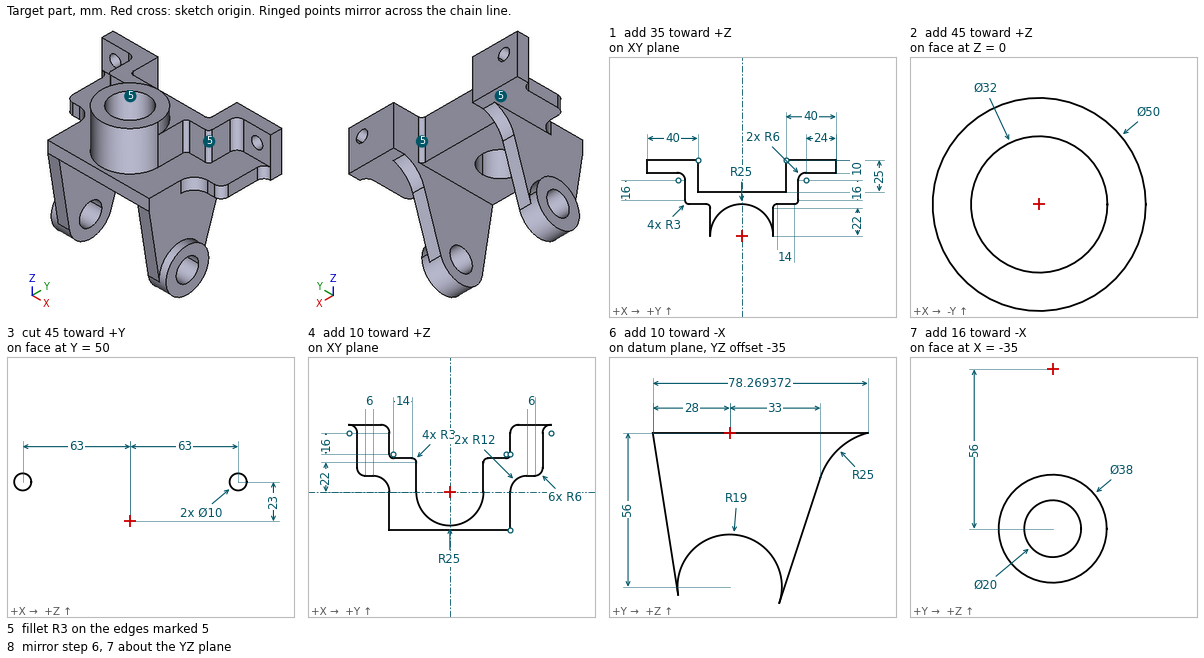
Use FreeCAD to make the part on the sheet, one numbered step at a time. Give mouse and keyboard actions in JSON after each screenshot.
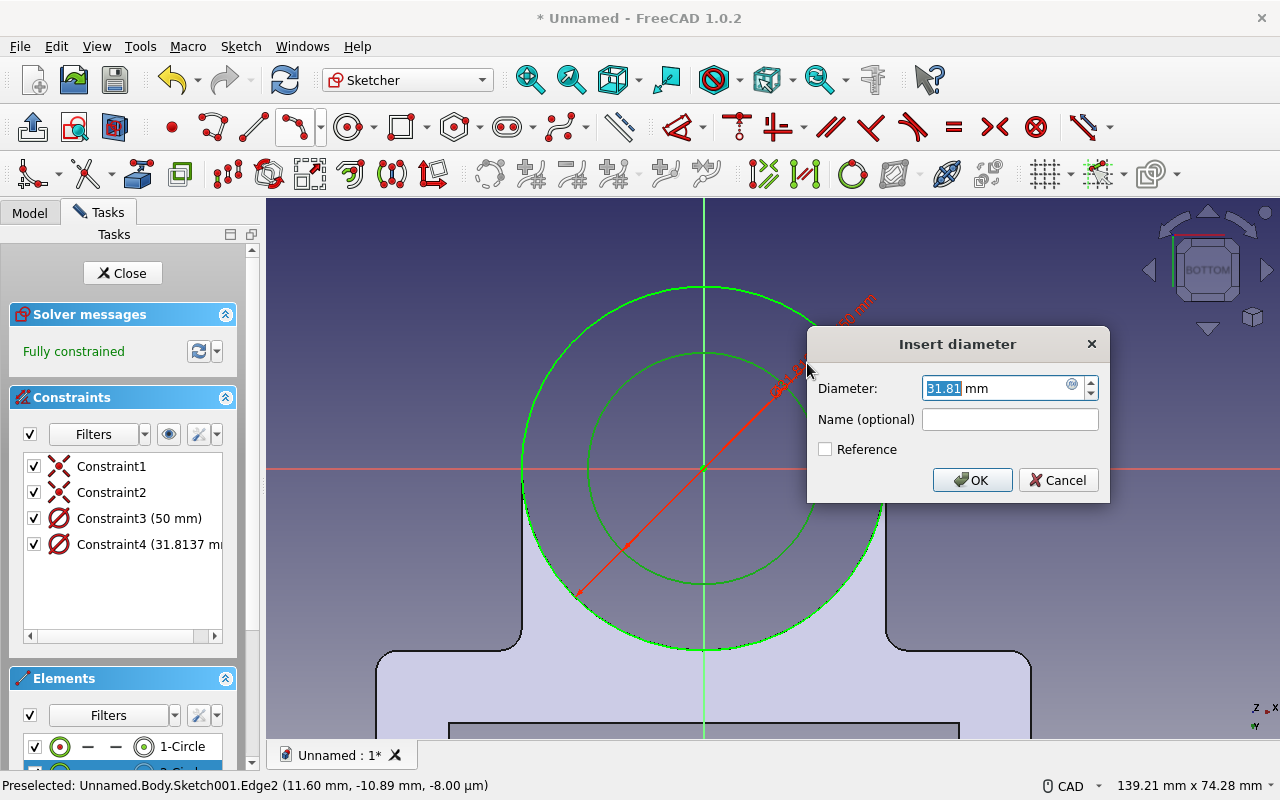
{"action": "type", "text": "32"}
{"action": "key", "text": "Return"}
{"action": "key", "text": "Escape"}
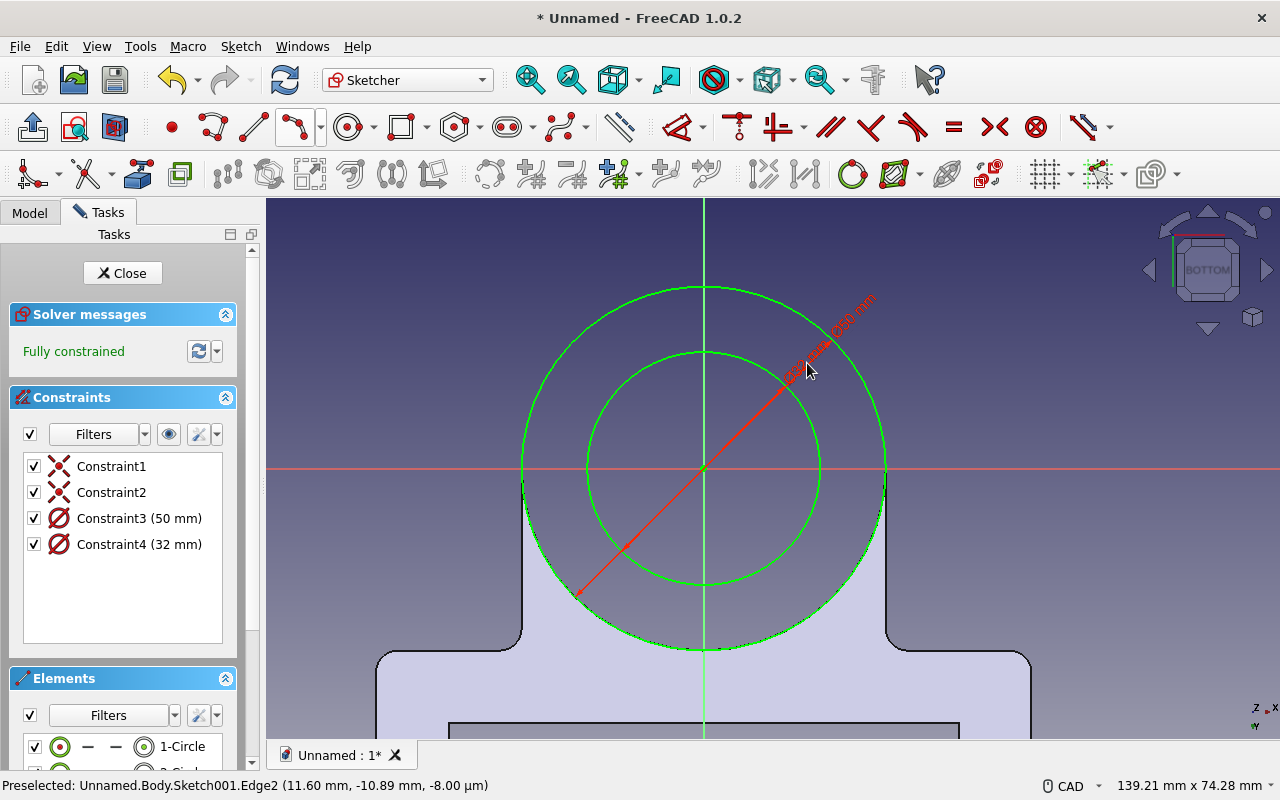
{"action": "left_click", "coordinate": [123, 273]}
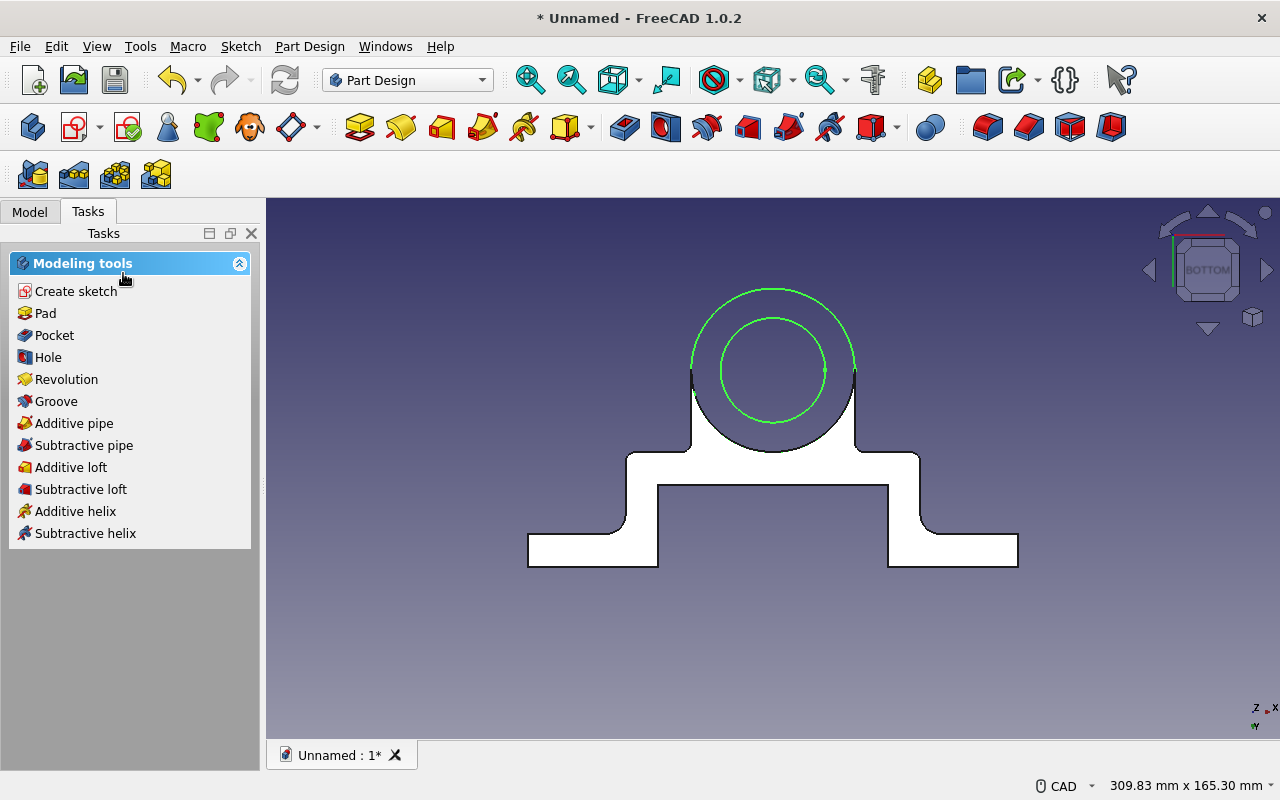
{"action": "left_click", "coordinate": [360, 128]}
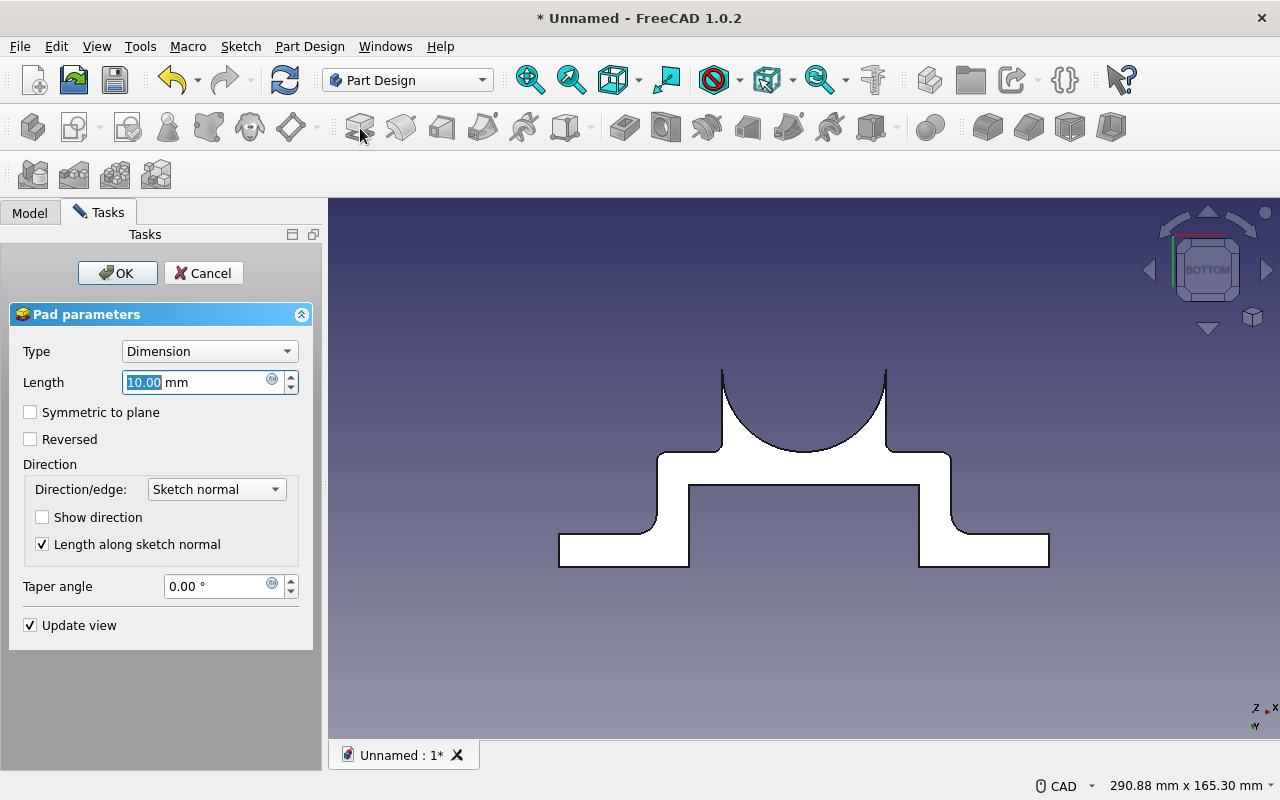
{"action": "type", "text": "45"}
{"action": "key", "text": "Tab"}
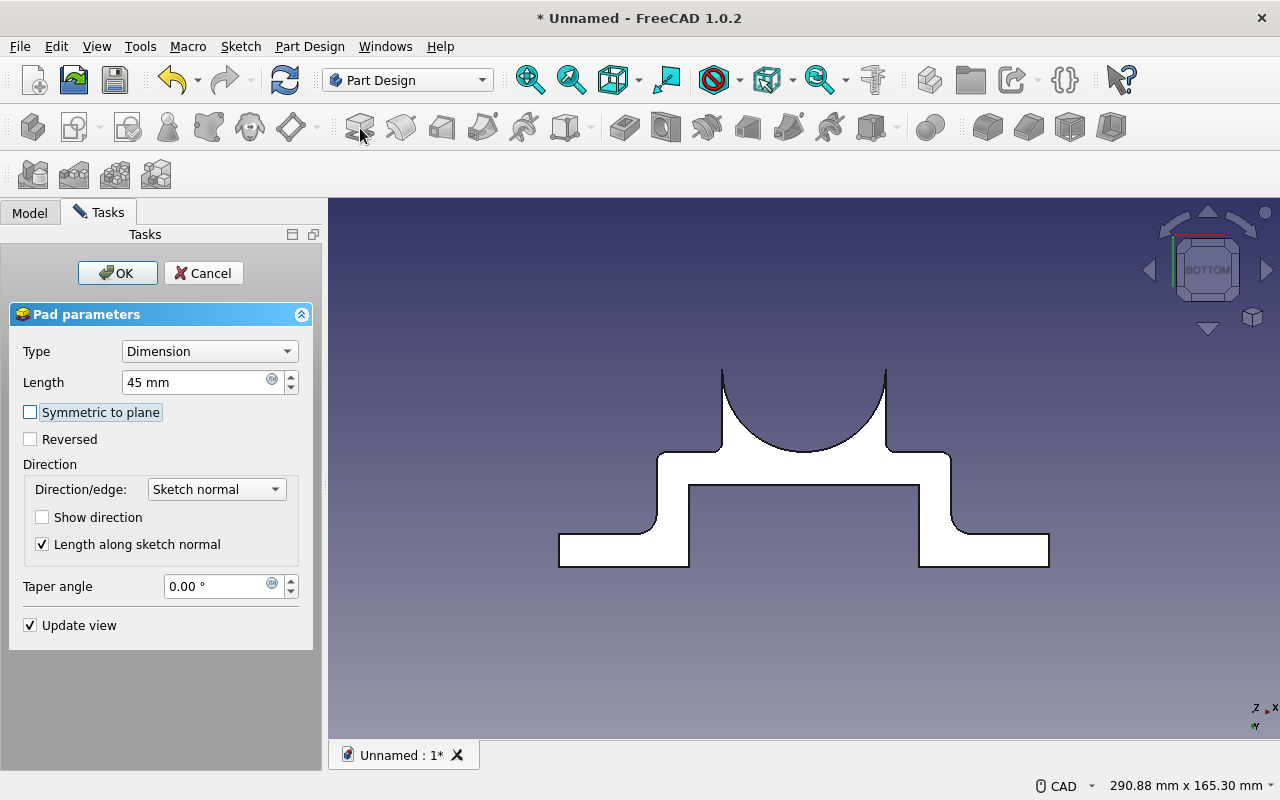
{"action": "left_click", "coordinate": [31, 439]}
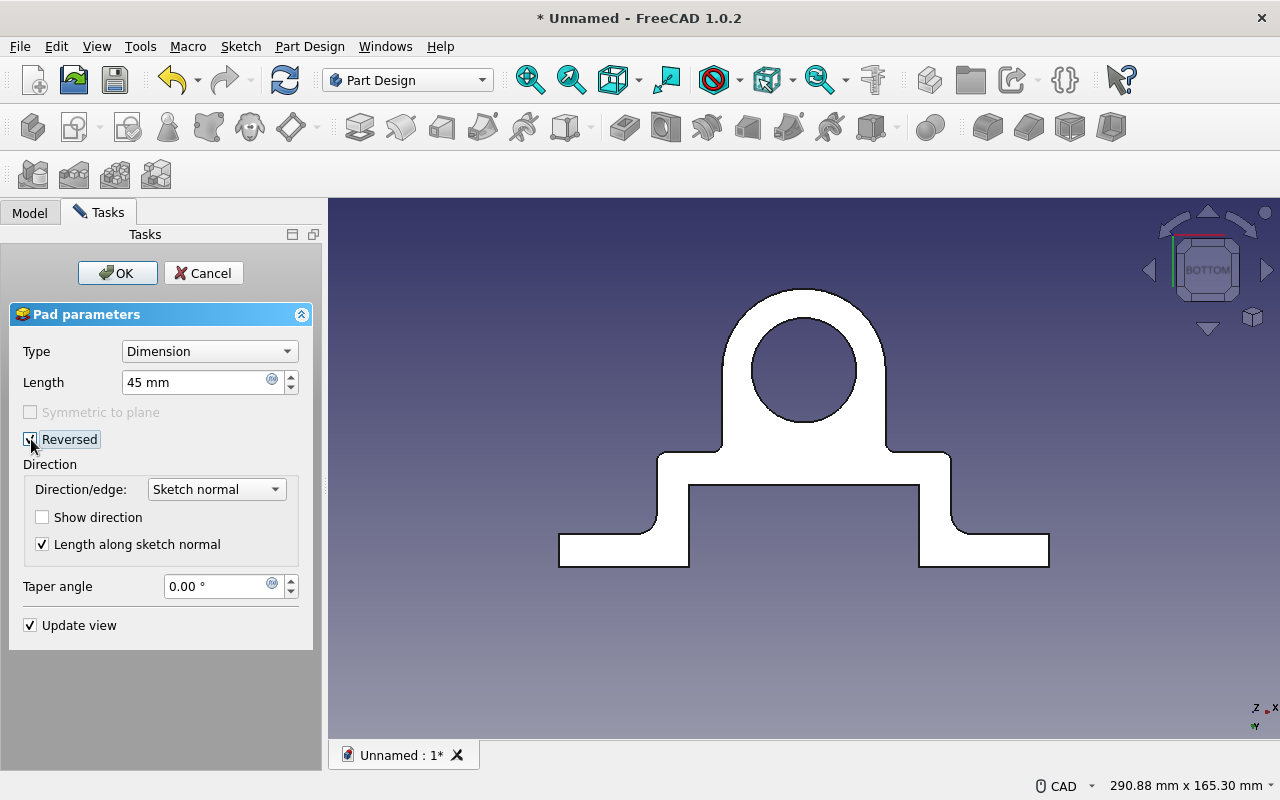
{"action": "left_click", "coordinate": [118, 273]}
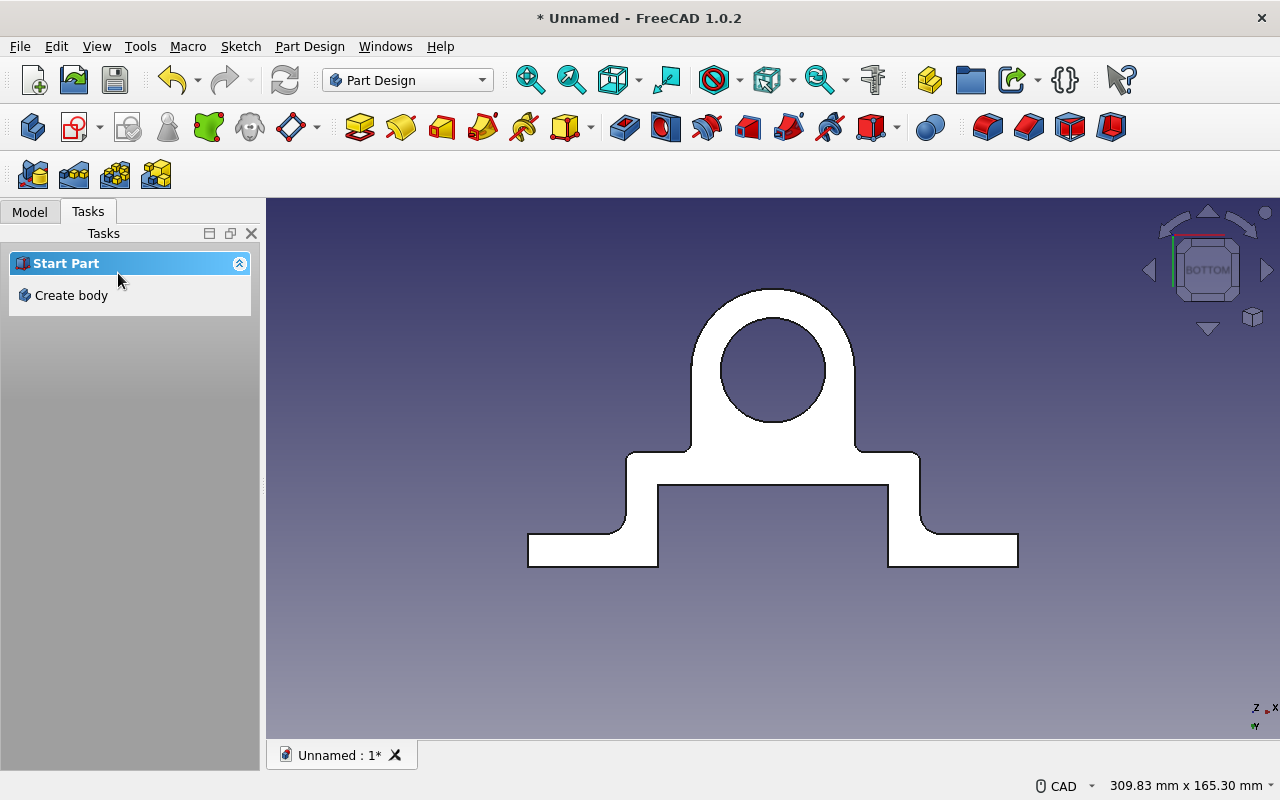
{"action": "key", "text": "0"}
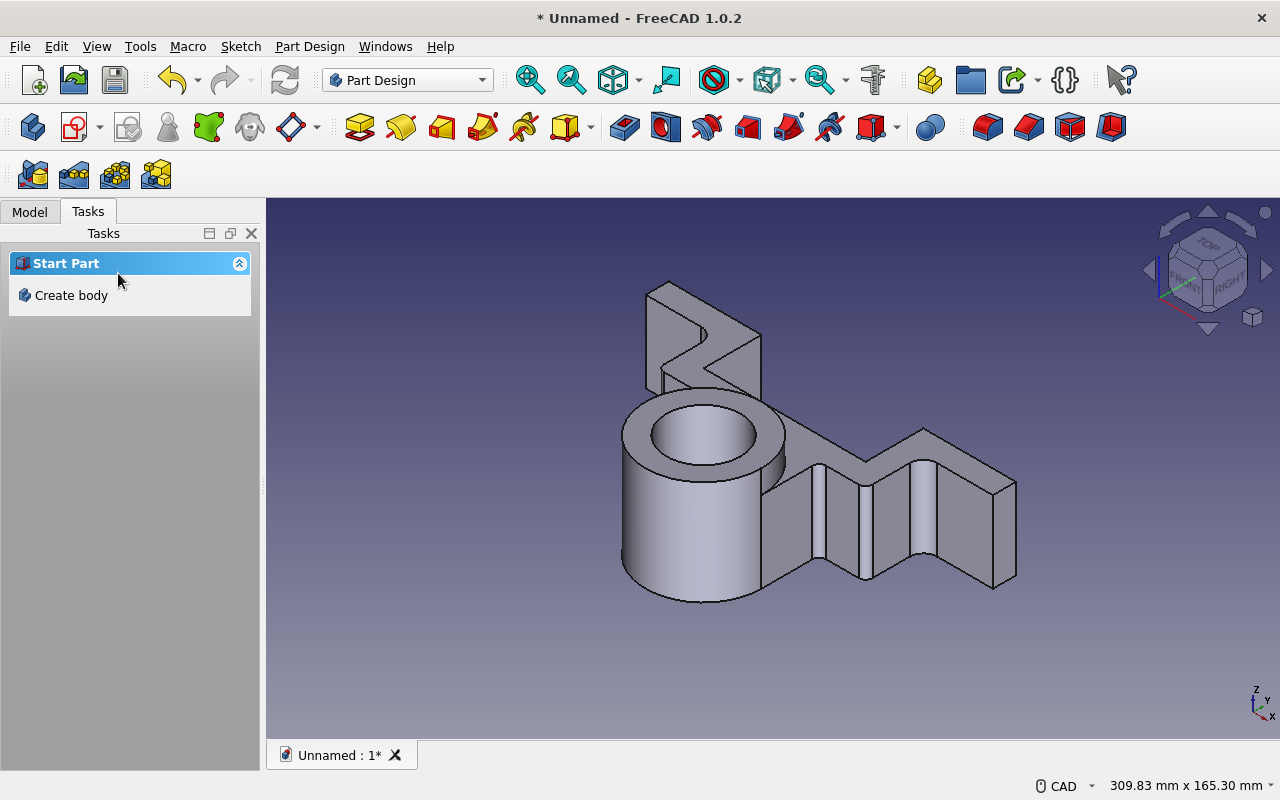
{"action": "left_click", "coordinate": [673, 343]}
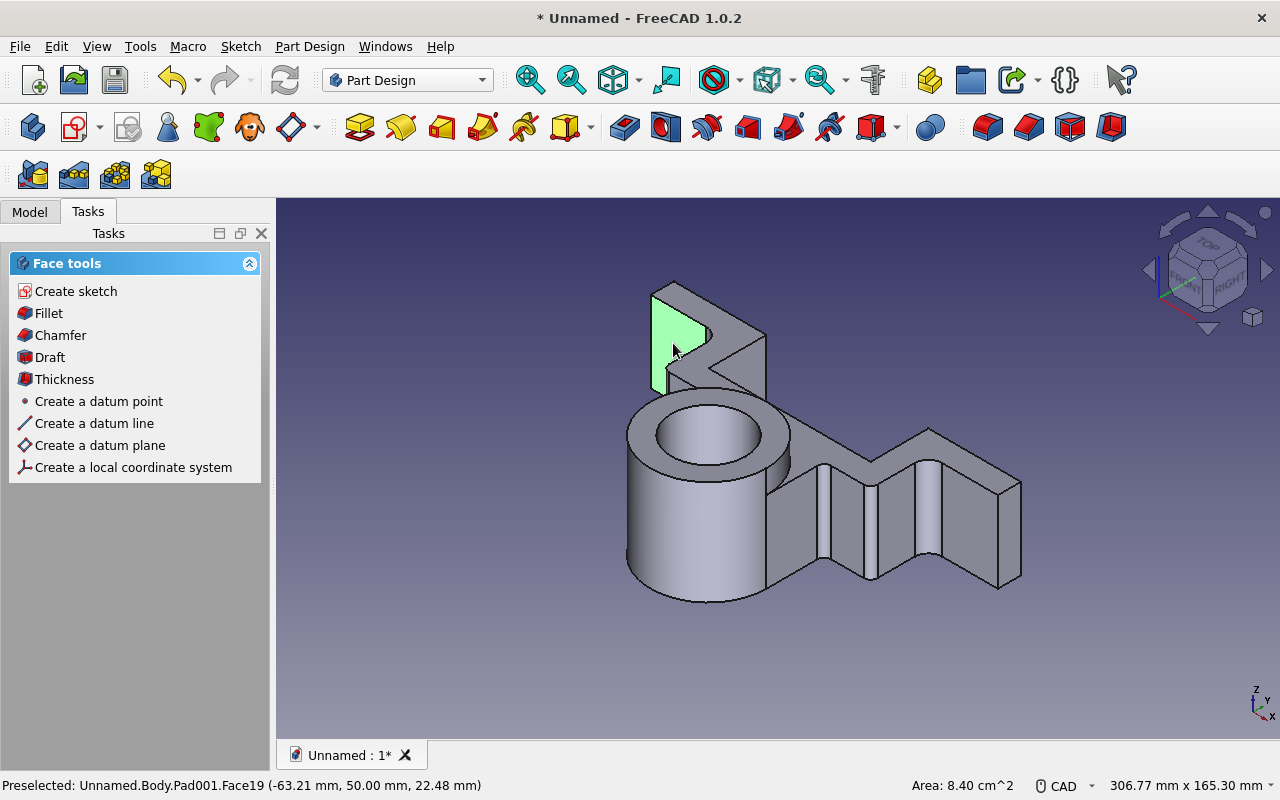
{"action": "left_click", "coordinate": [74, 128]}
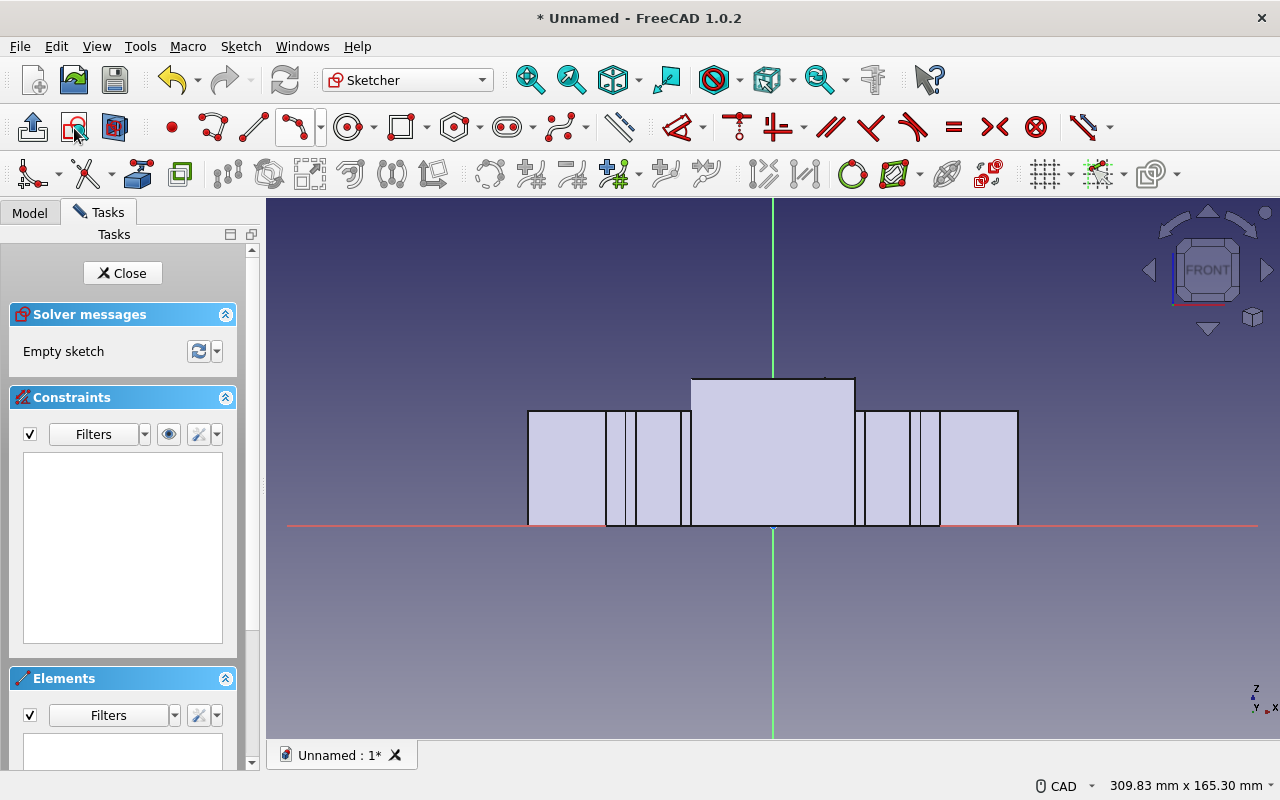
{"action": "left_click", "coordinate": [115, 128]}